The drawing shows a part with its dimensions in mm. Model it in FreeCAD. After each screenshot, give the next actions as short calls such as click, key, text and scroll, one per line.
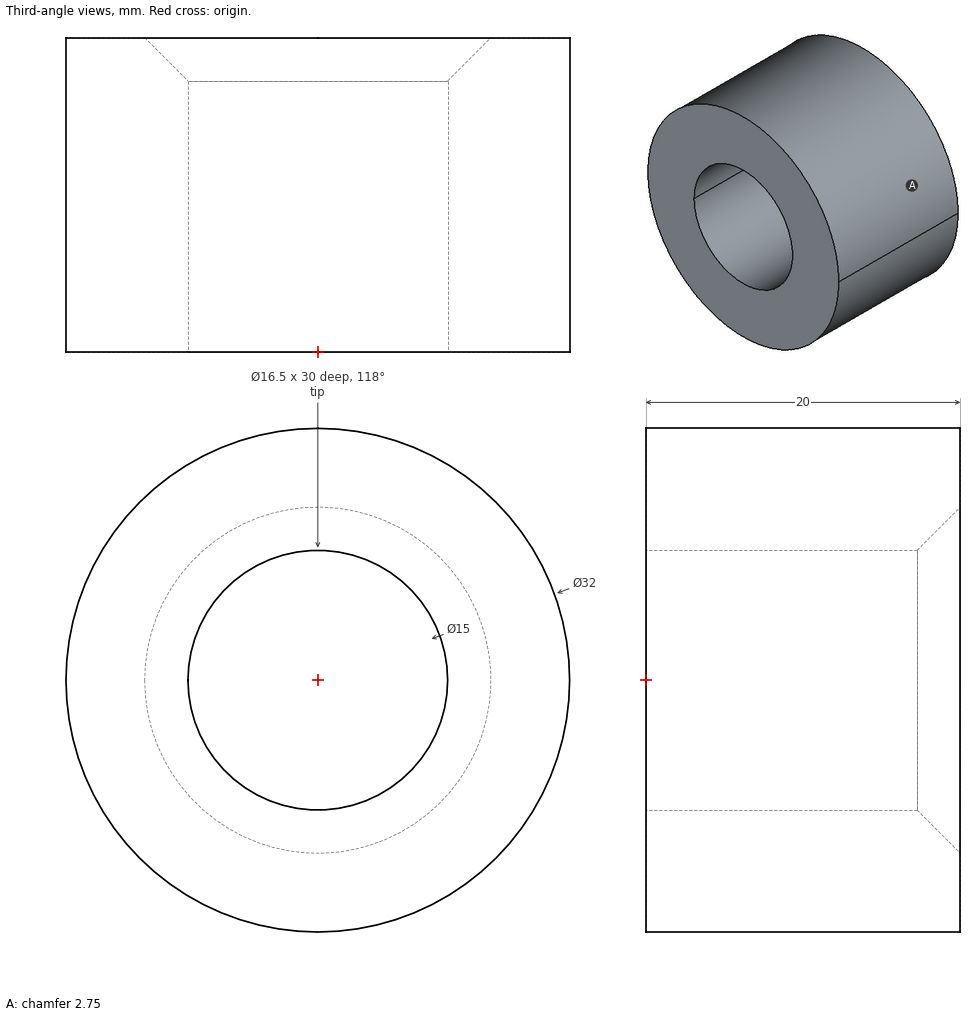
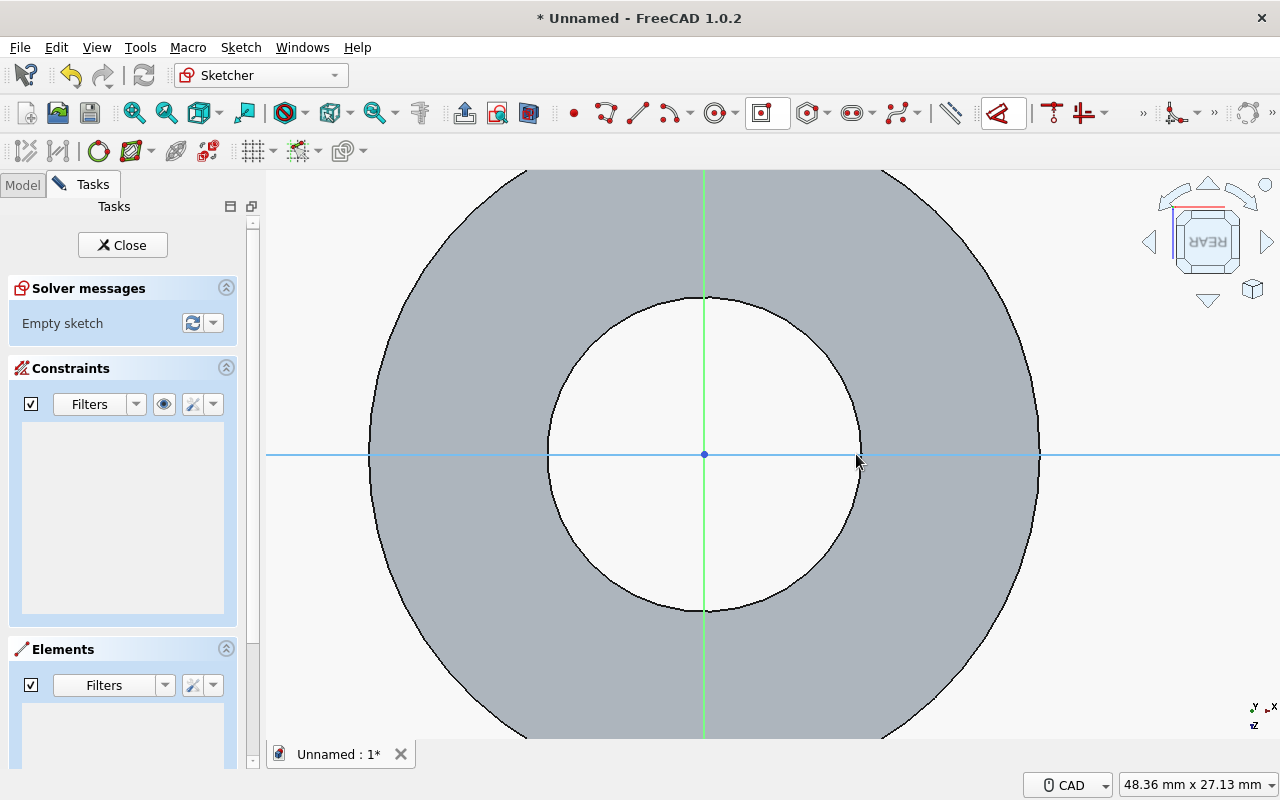
key(g)
key(c)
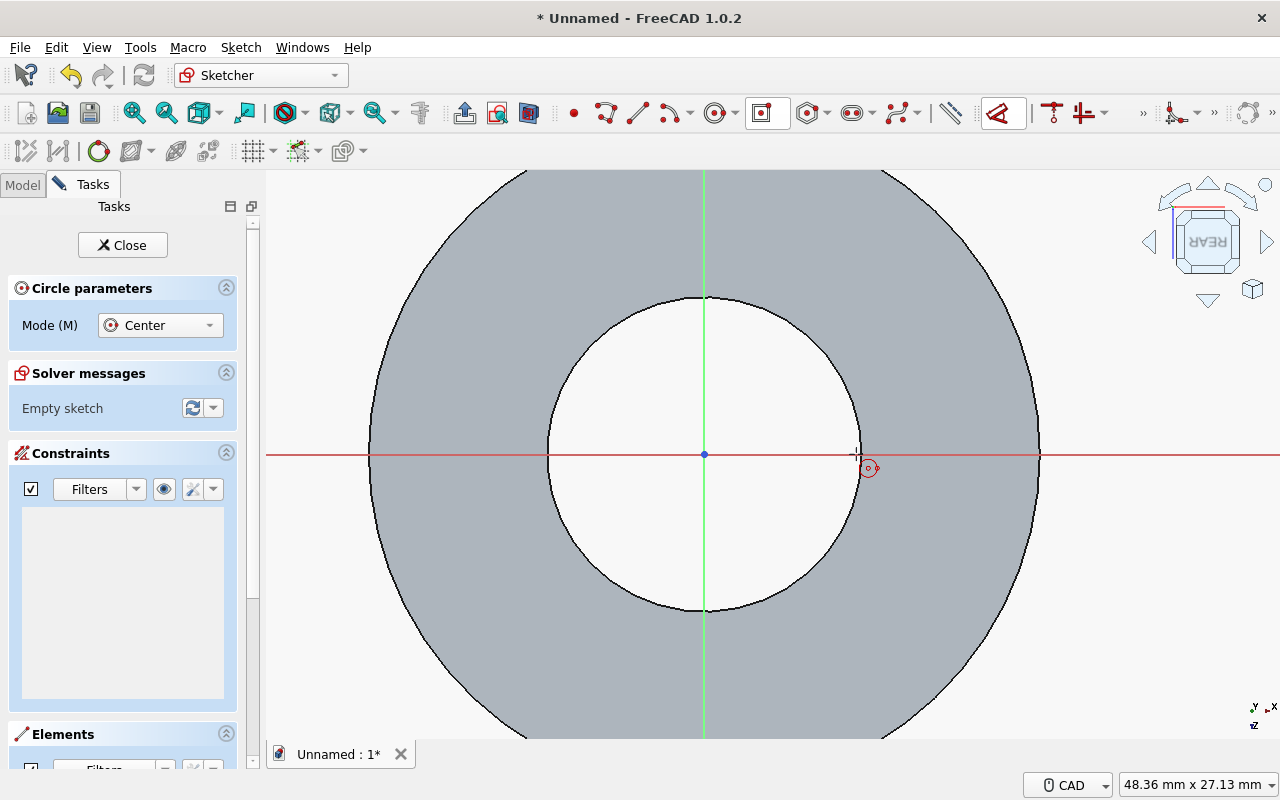
click(704, 454)
move(827, 332)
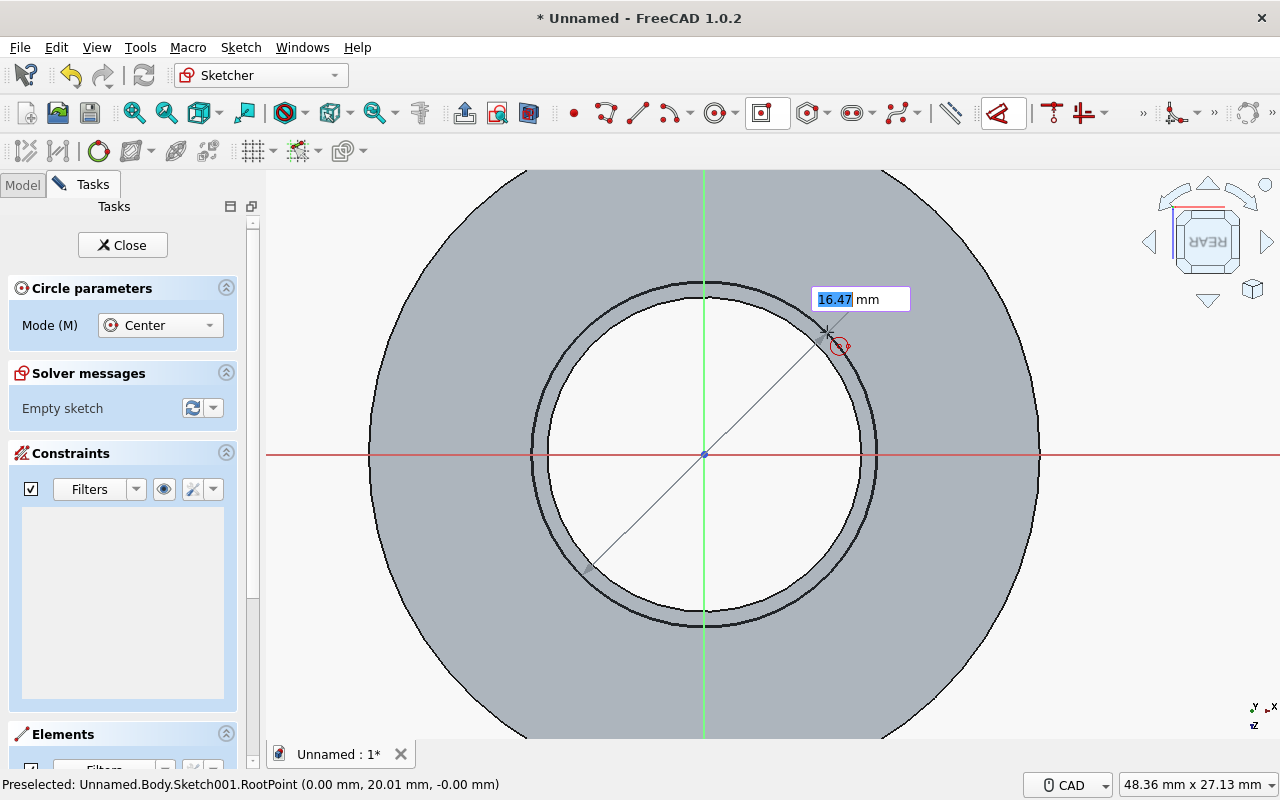
text(16.5)
key(Return)
key(Escape)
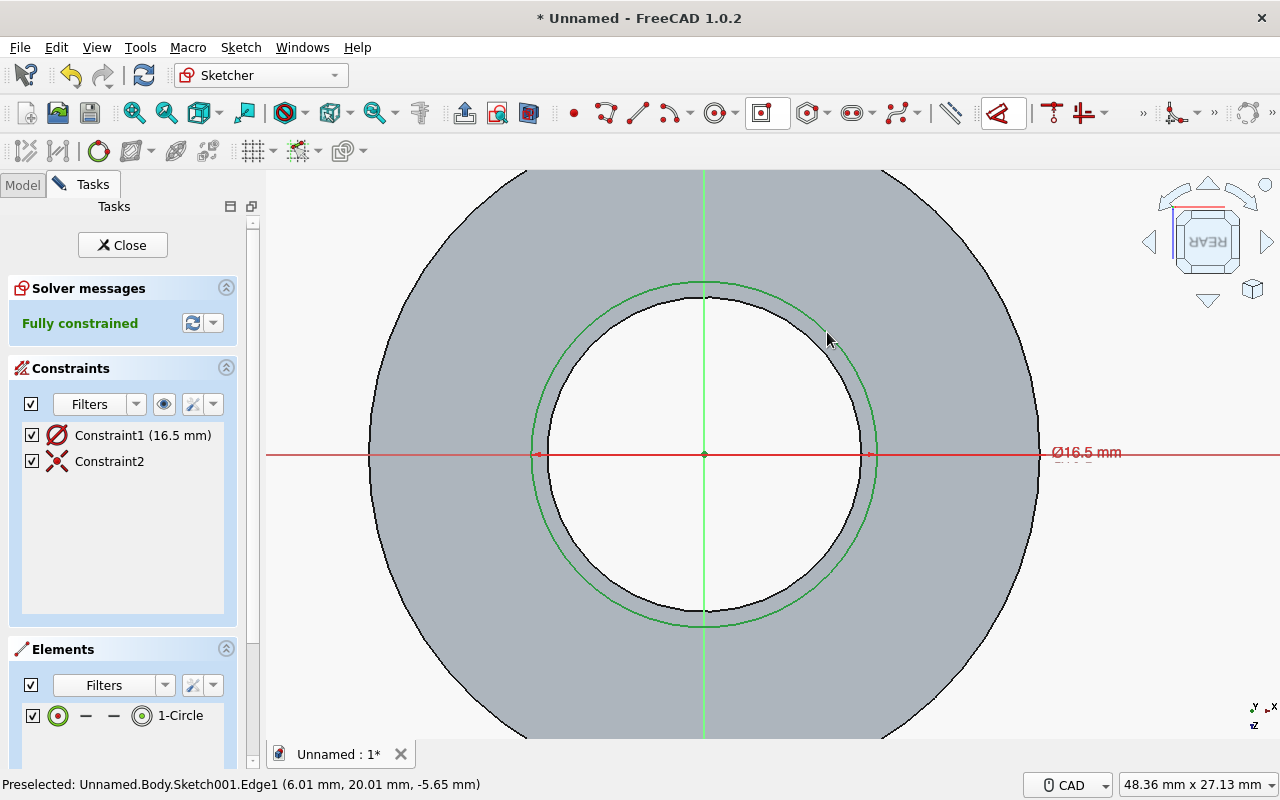
click(123, 245)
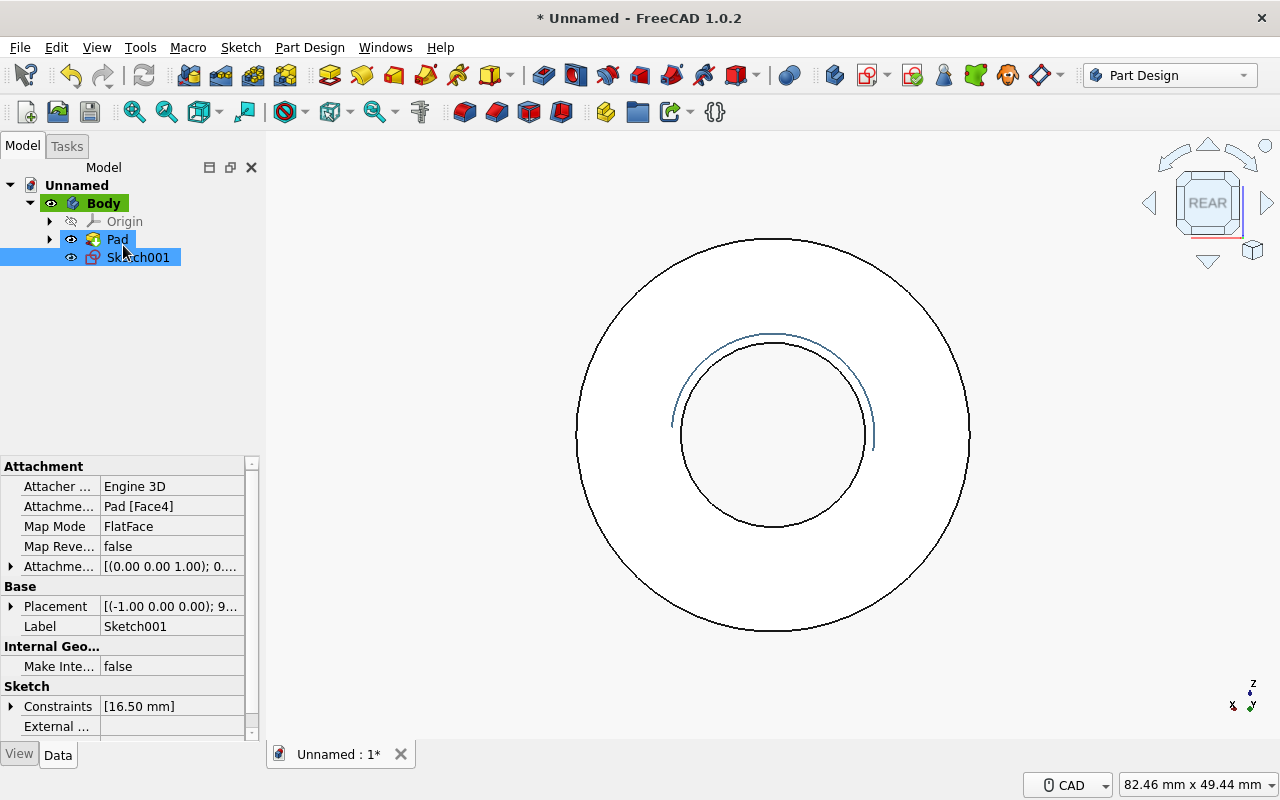
click(576, 76)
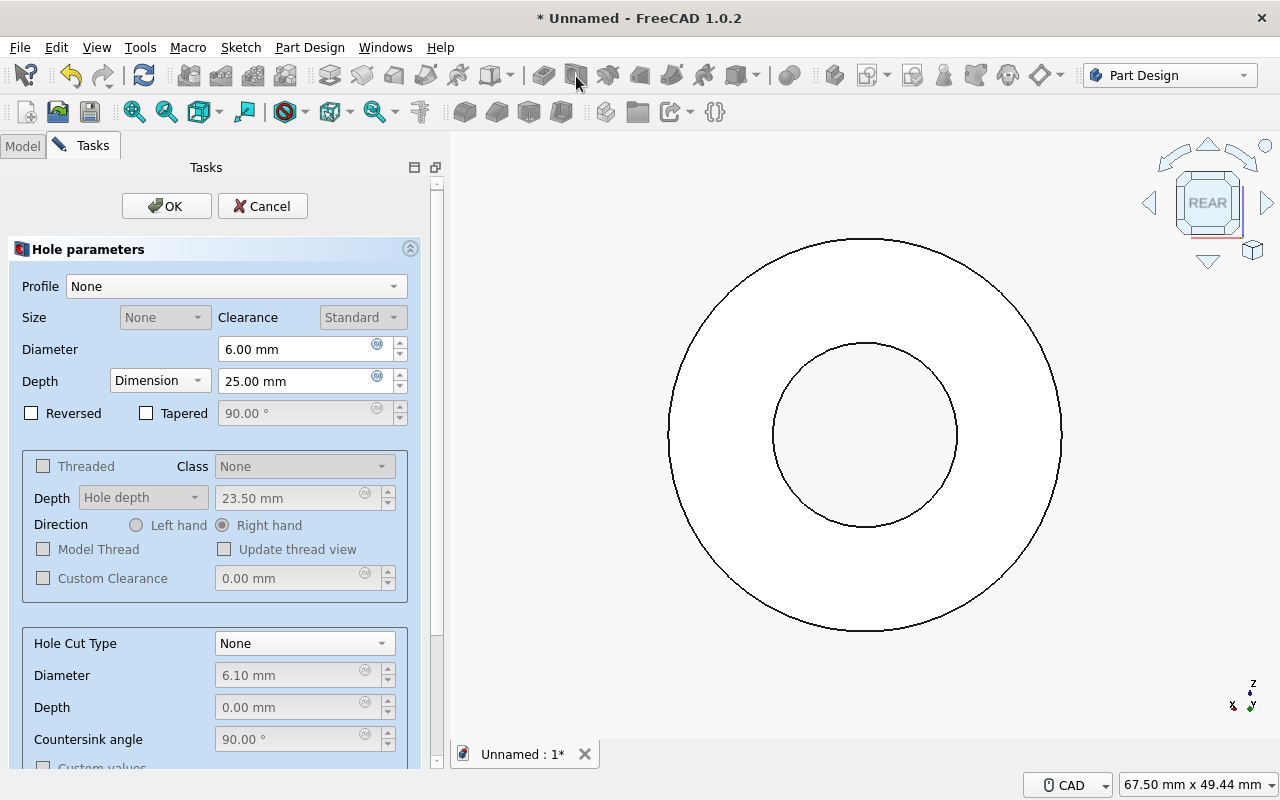
triple_click(305, 349)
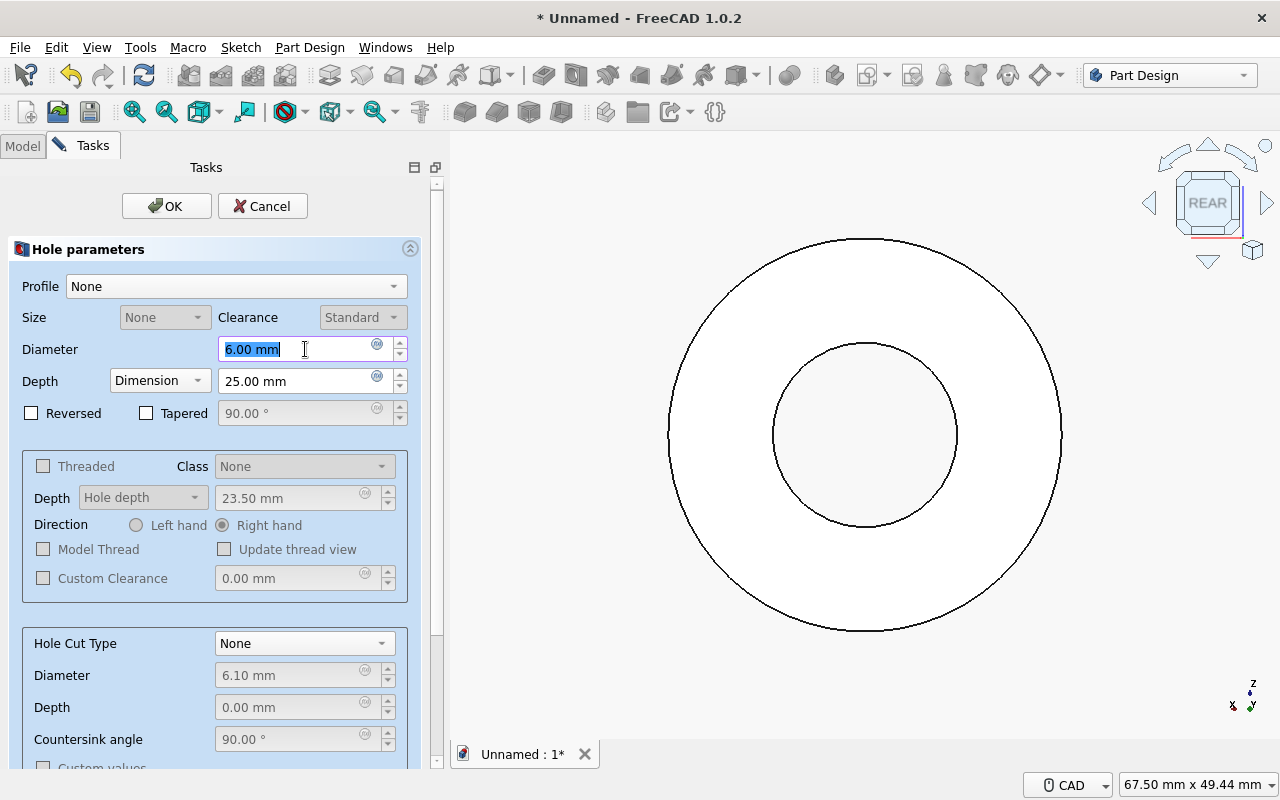
text(16.5)
key(Tab)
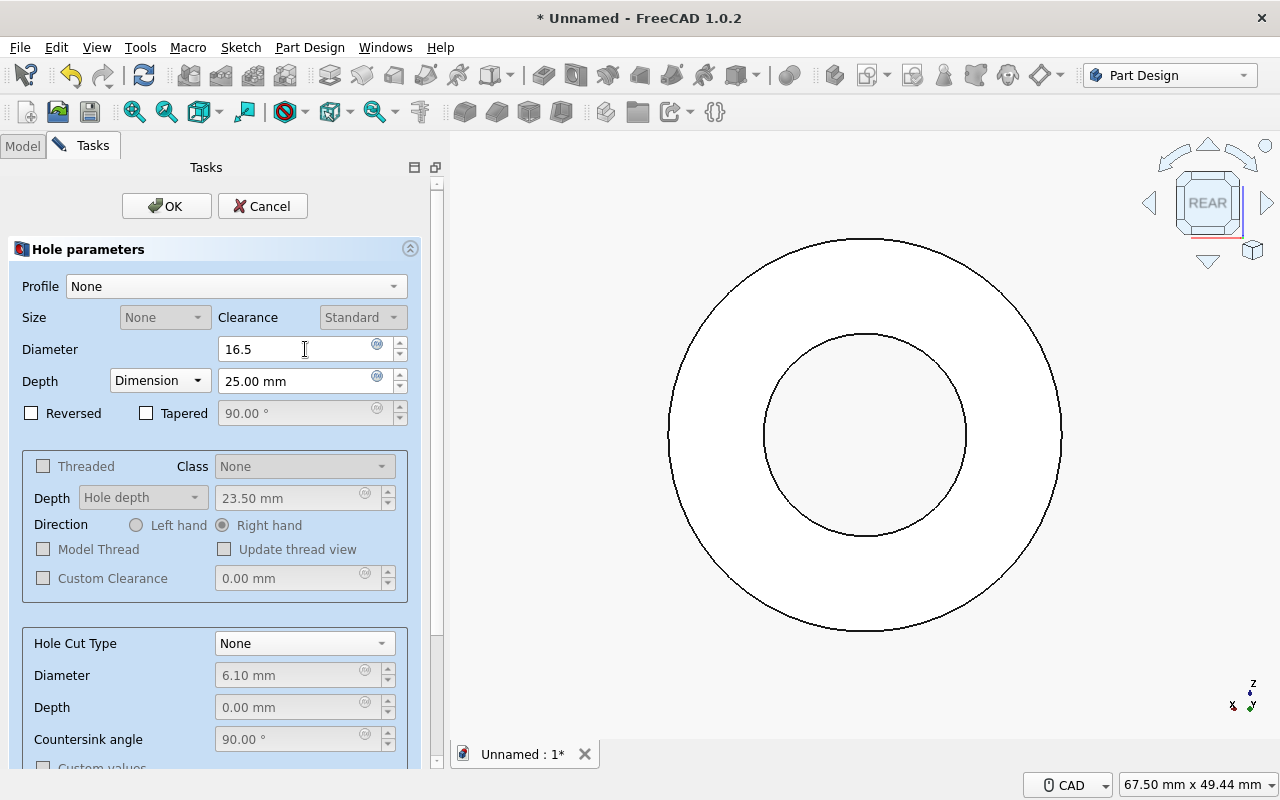
triple_click(305, 381)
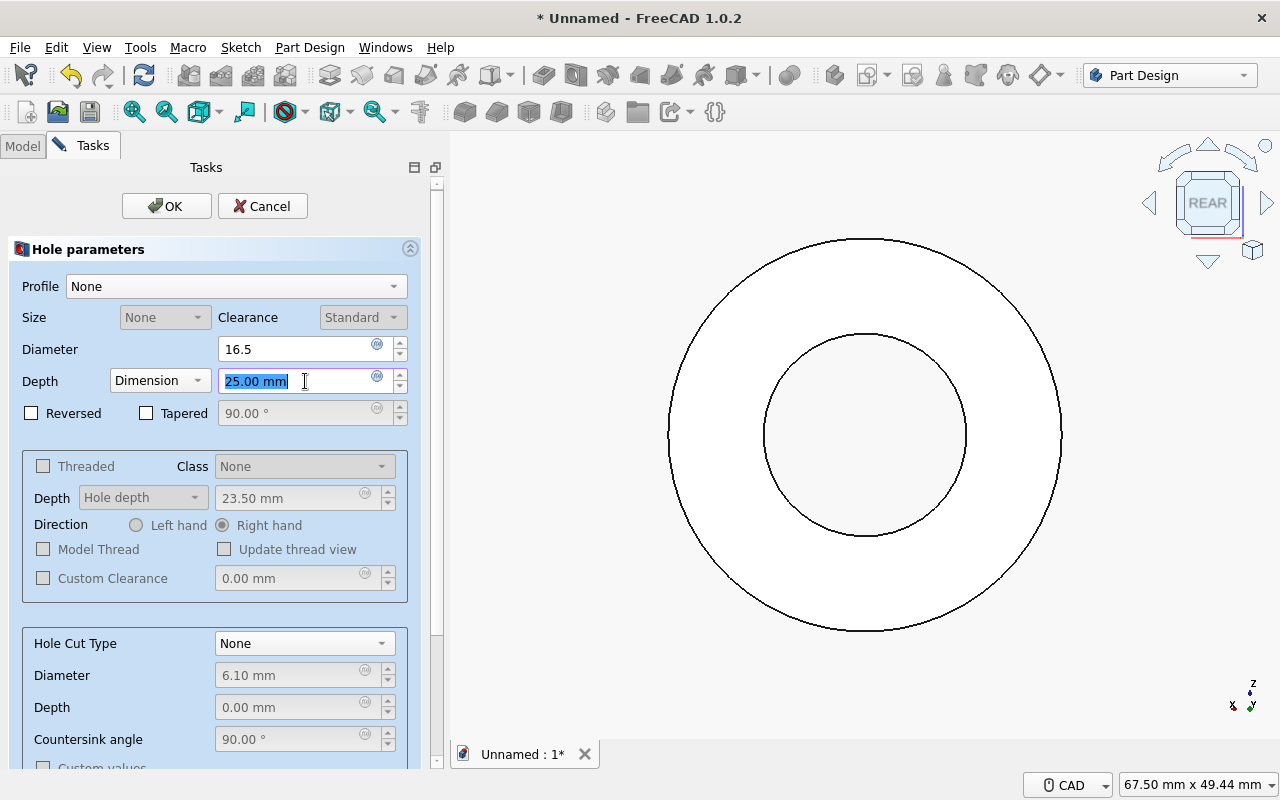
text(30)
key(Tab)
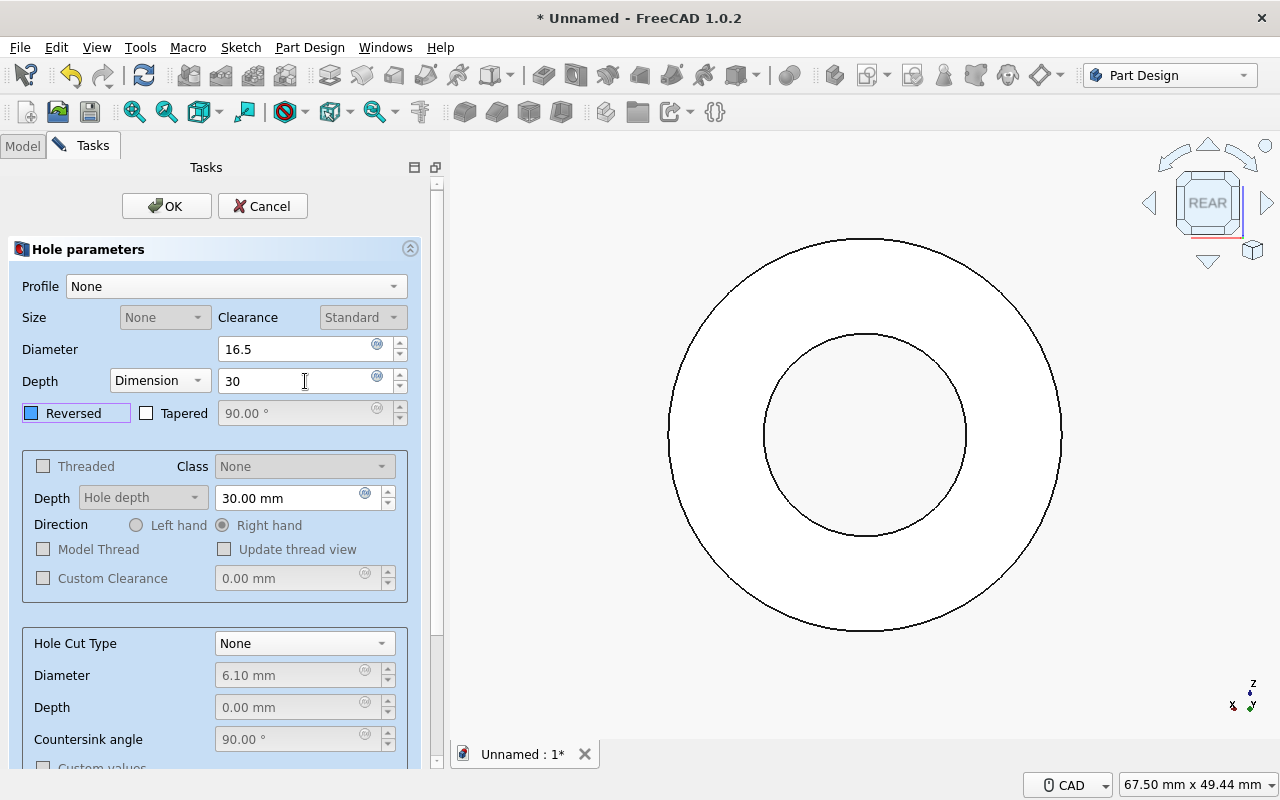
click(167, 206)